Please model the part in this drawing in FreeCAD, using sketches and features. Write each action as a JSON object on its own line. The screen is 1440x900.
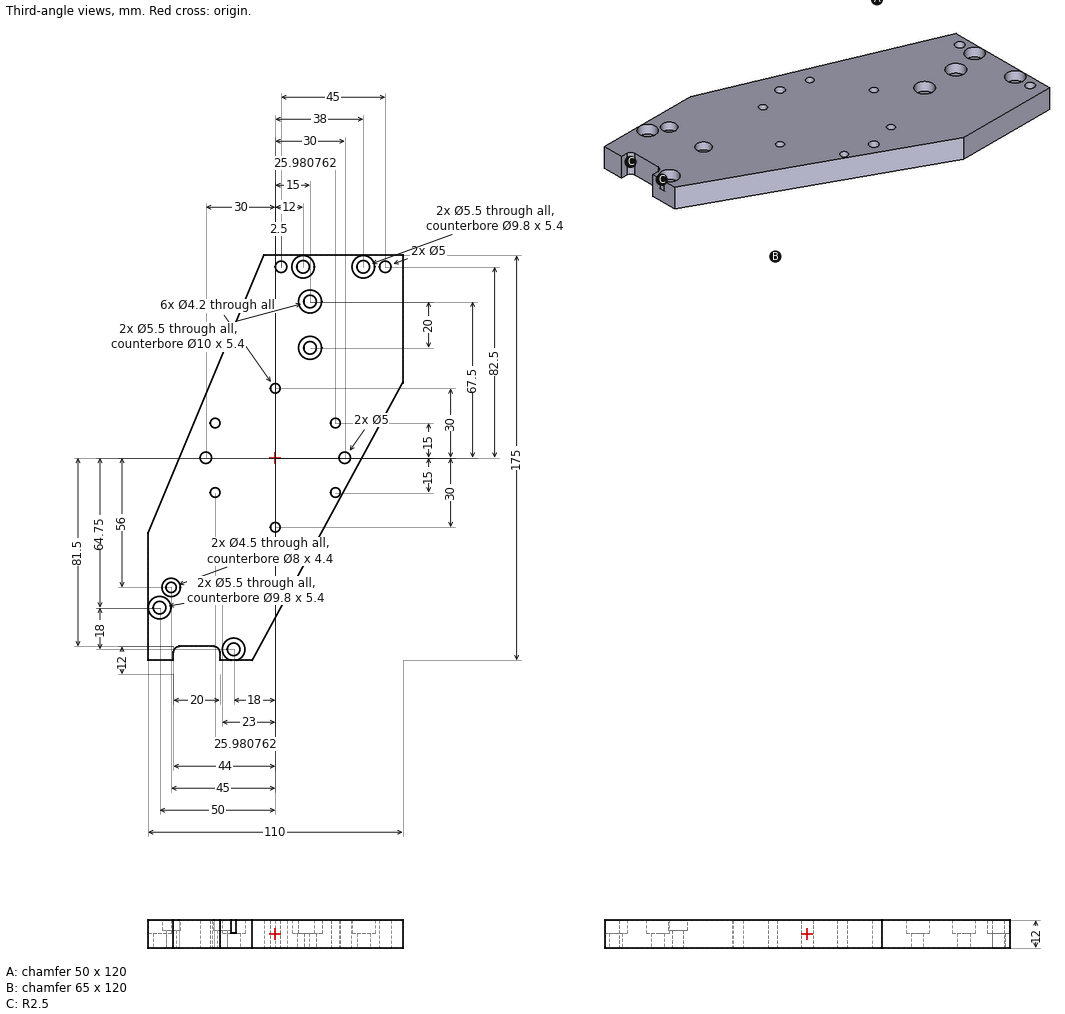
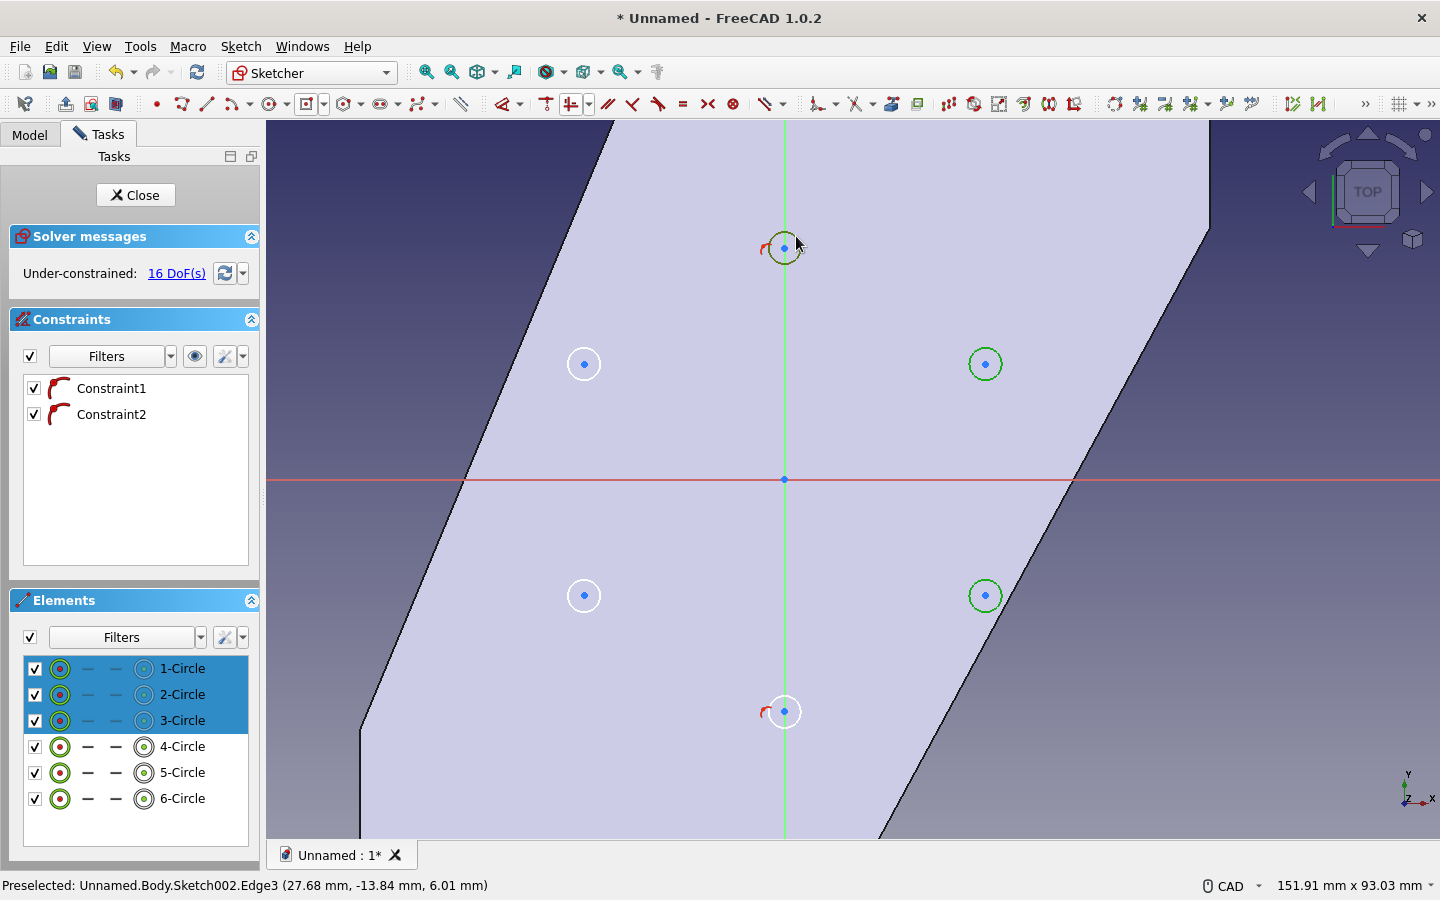
{"action": "scroll", "coordinate": [796, 701], "scroll_direction": "up", "scroll_amount": 2}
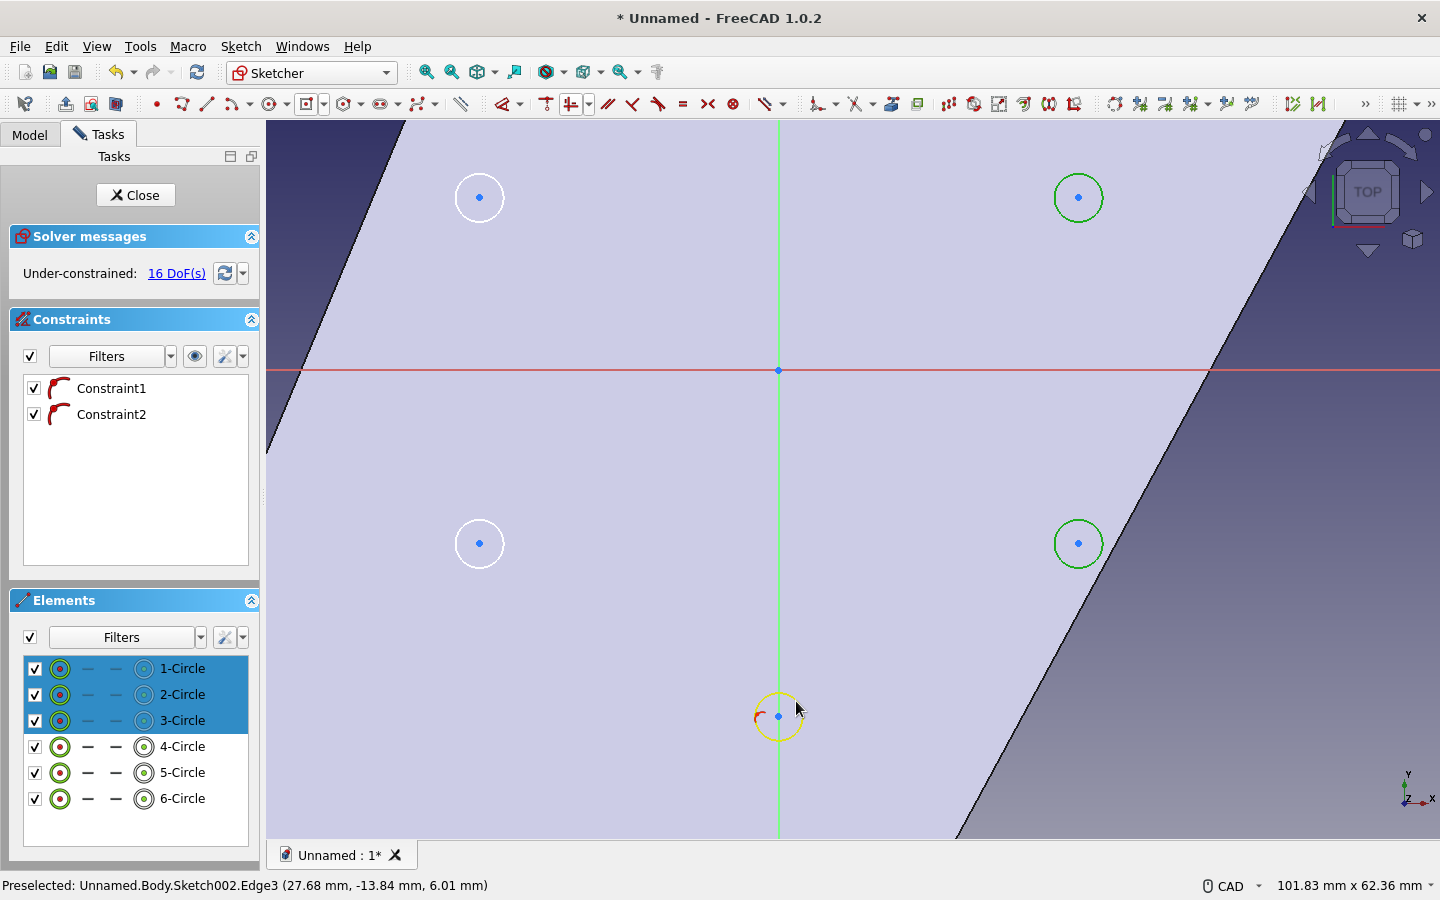
{"action": "left_click", "coordinate": [796, 700]}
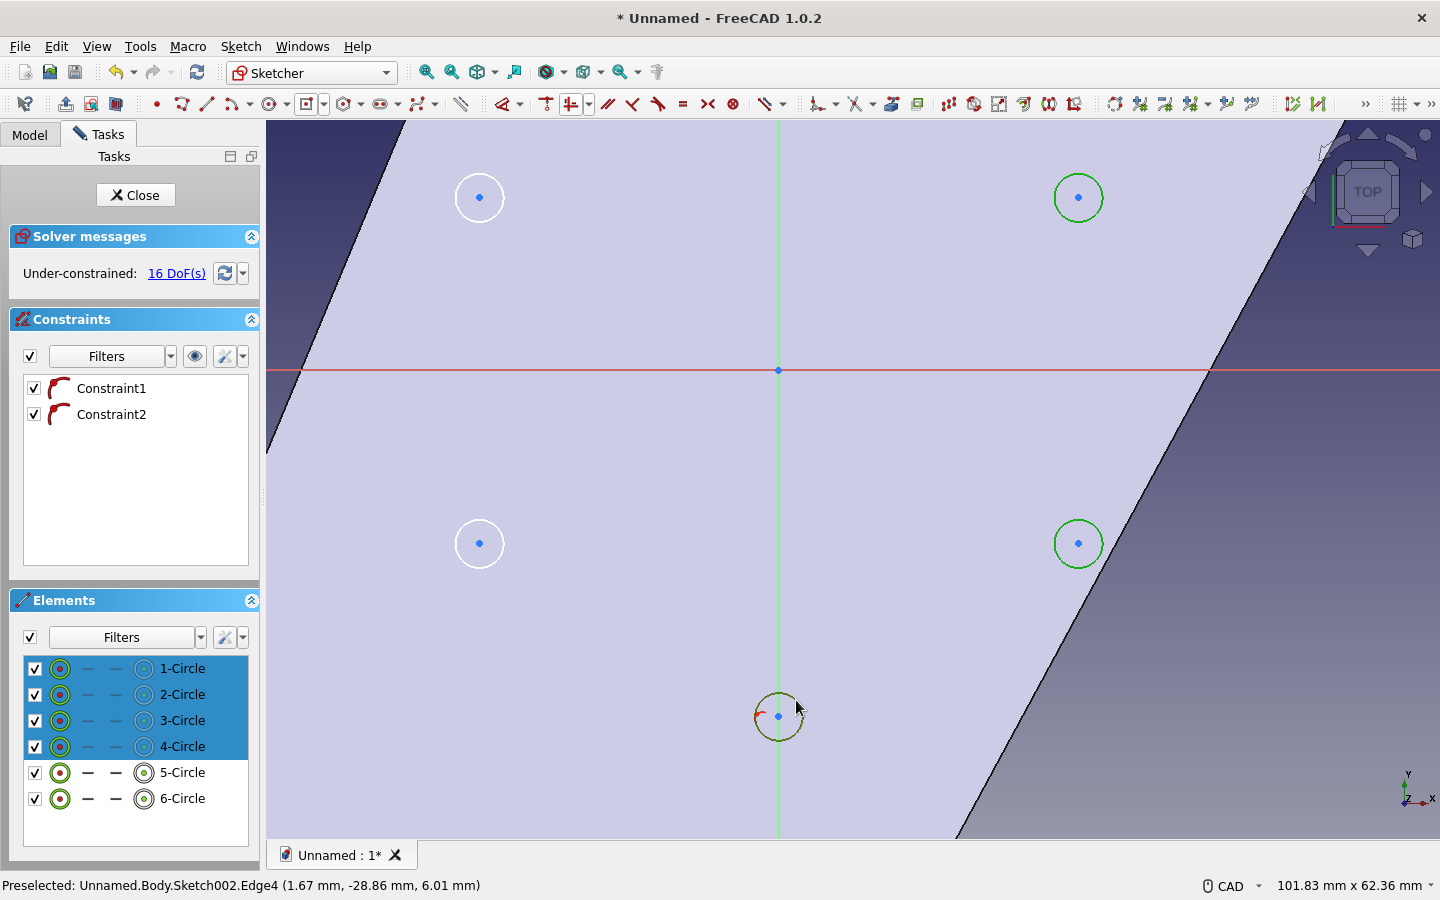
{"action": "left_click", "coordinate": [497, 527]}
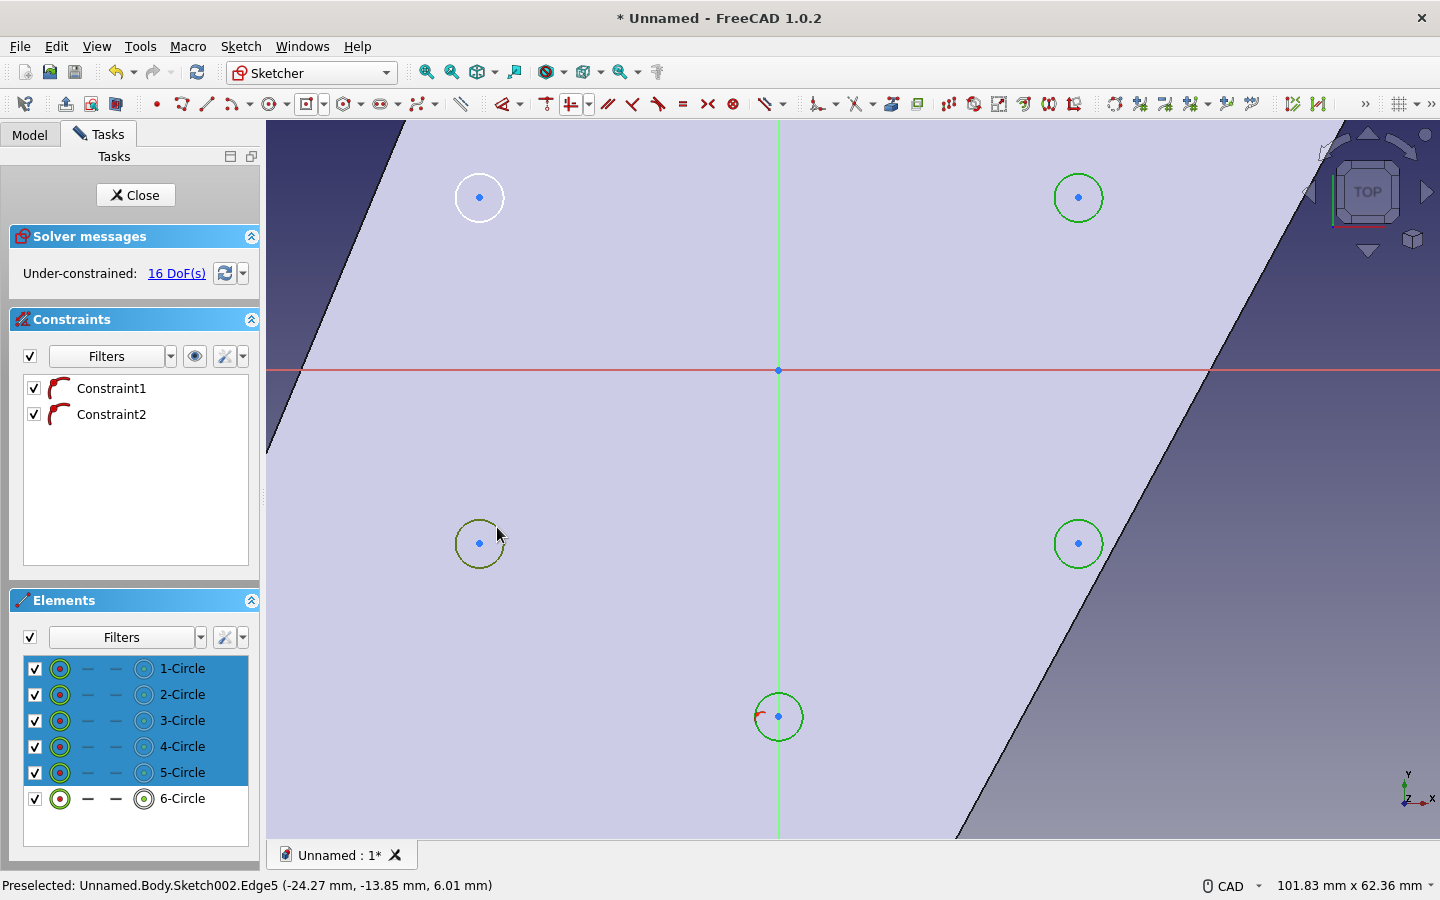
{"action": "left_click", "coordinate": [497, 181]}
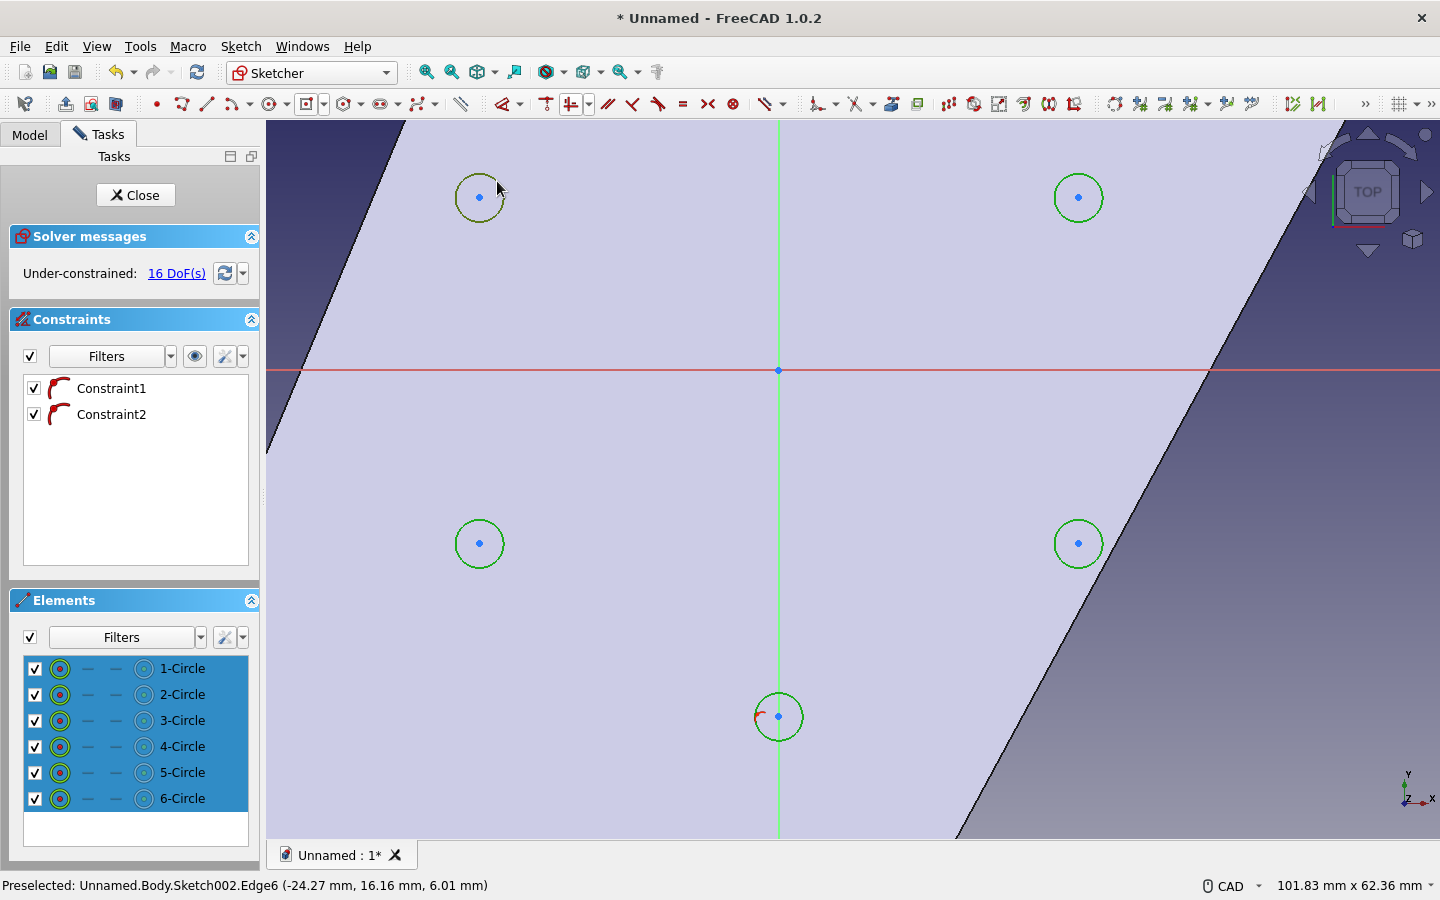
{"action": "key", "text": "e"}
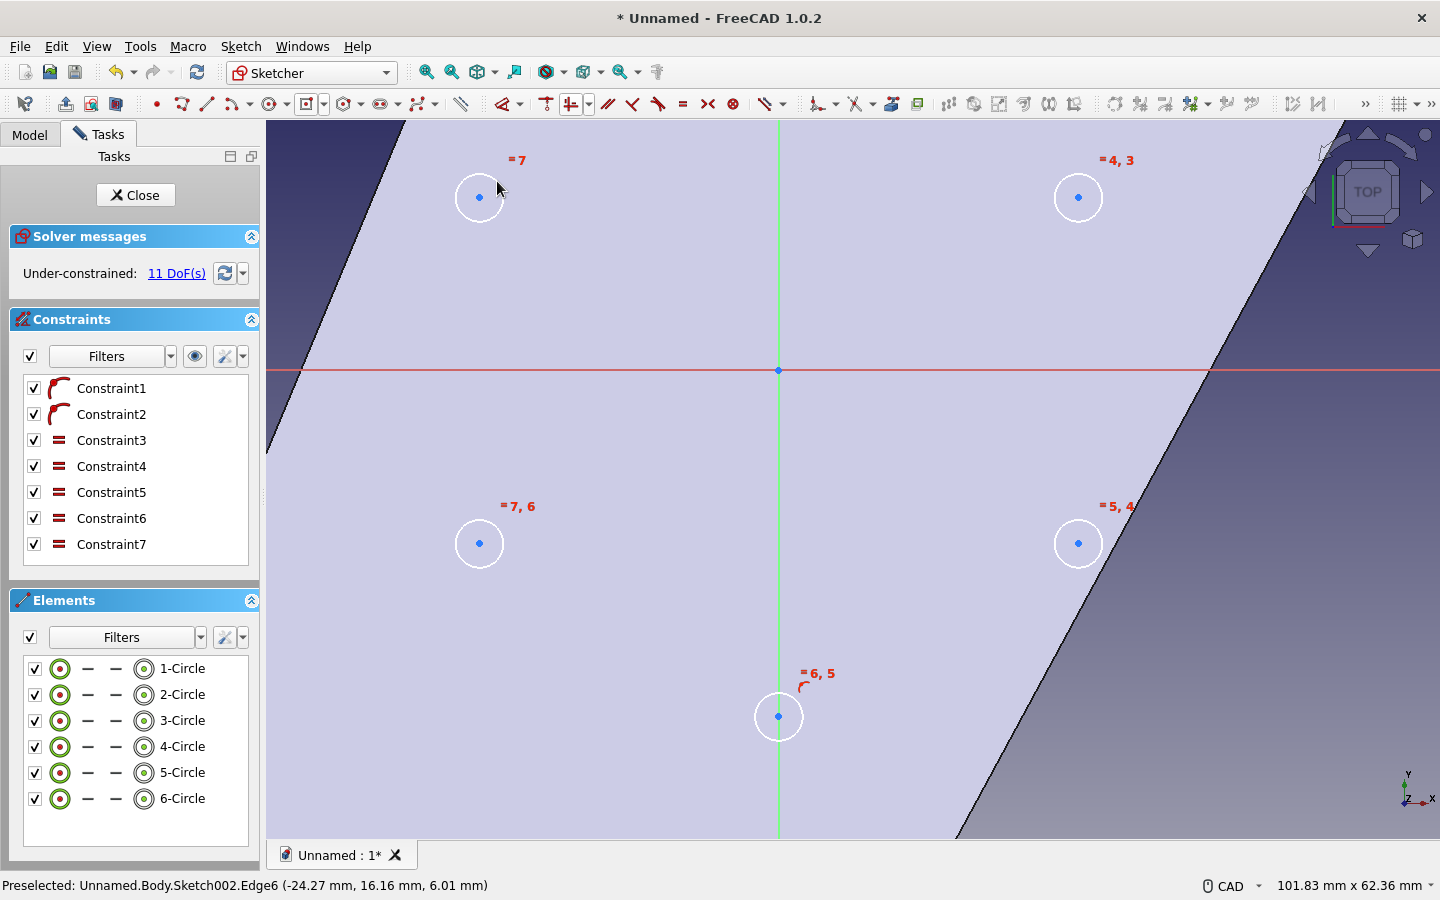
{"action": "left_click", "coordinate": [1079, 198]}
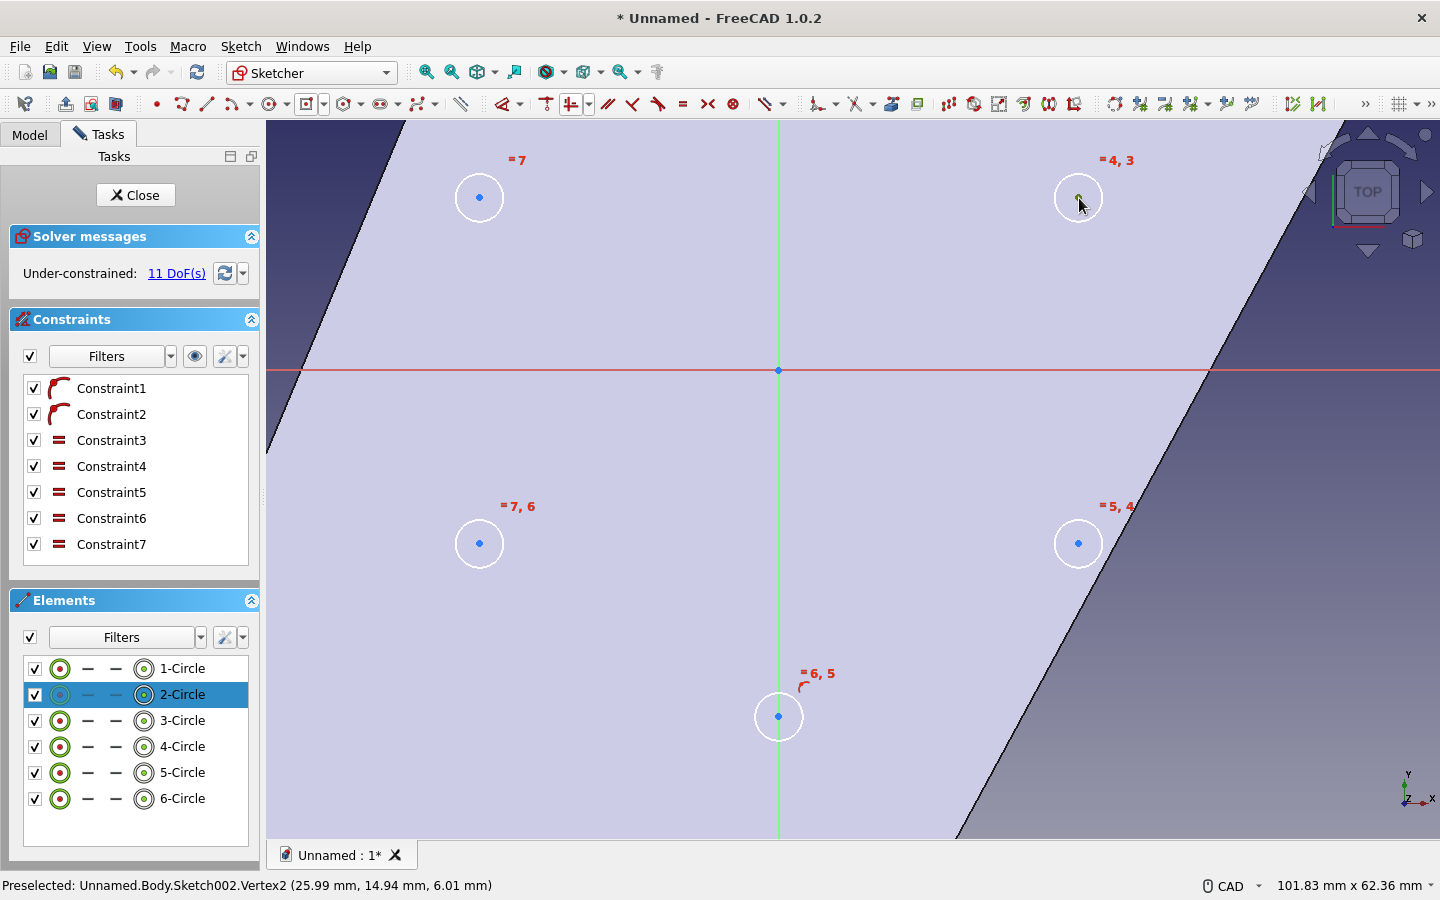
{"action": "left_click", "coordinate": [1079, 544]}